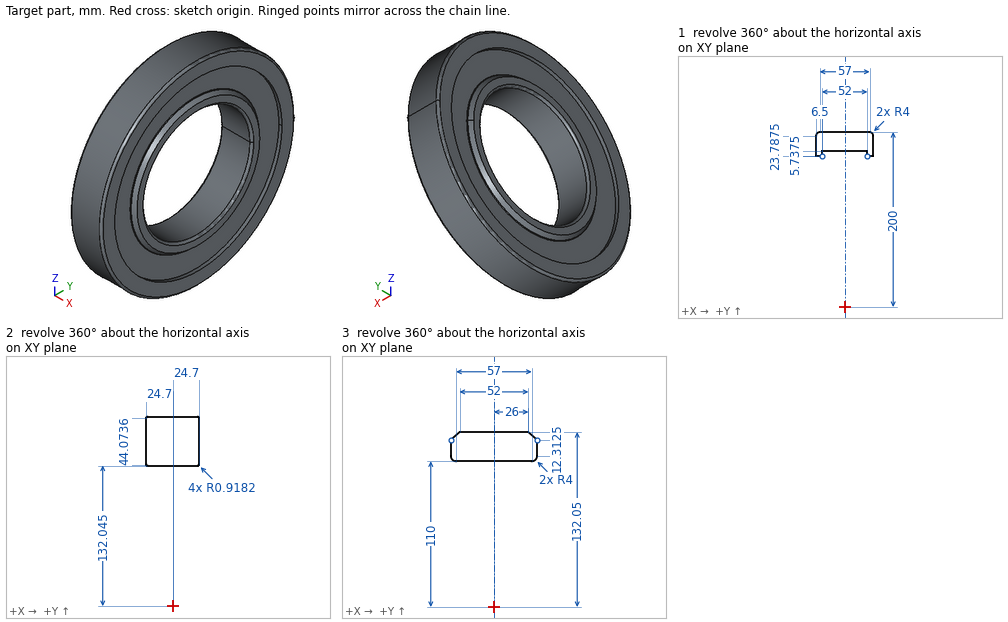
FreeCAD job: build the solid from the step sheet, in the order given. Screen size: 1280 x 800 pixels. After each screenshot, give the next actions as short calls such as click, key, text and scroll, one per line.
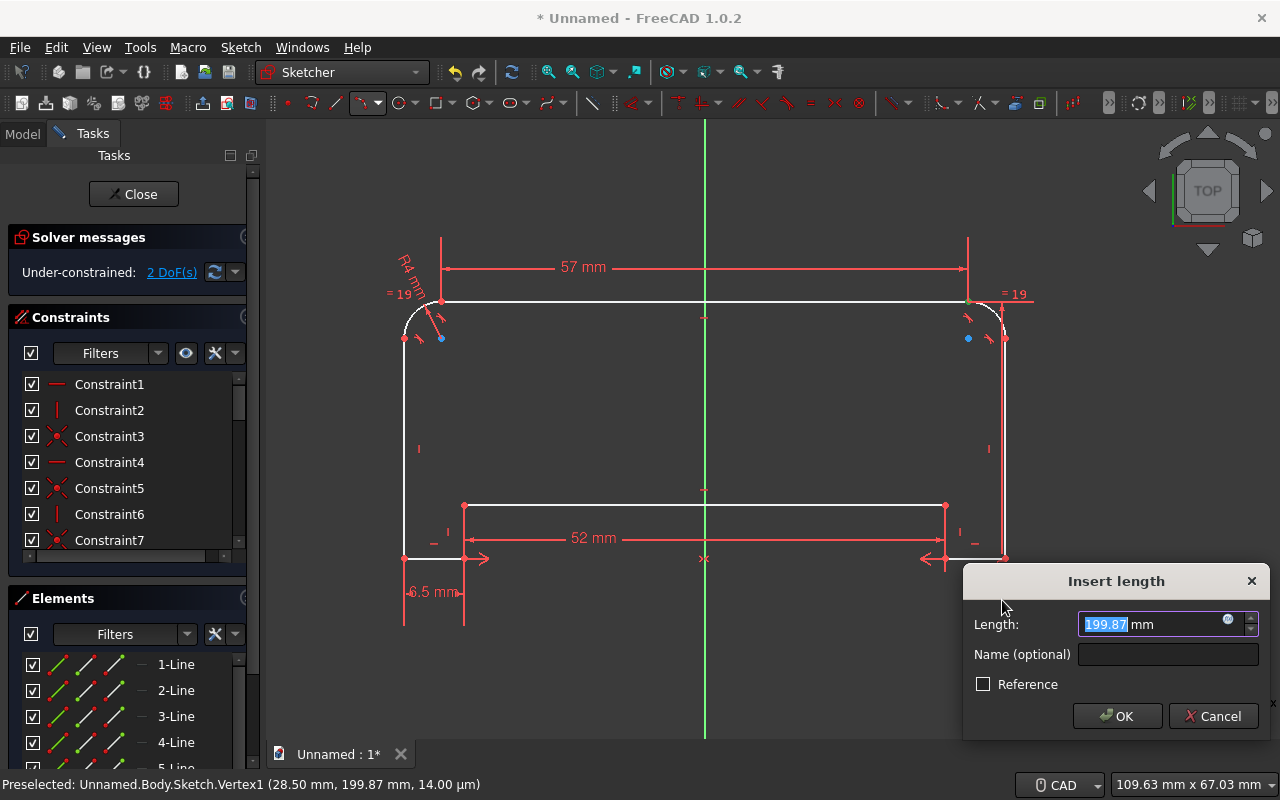
text(200)
key(Return)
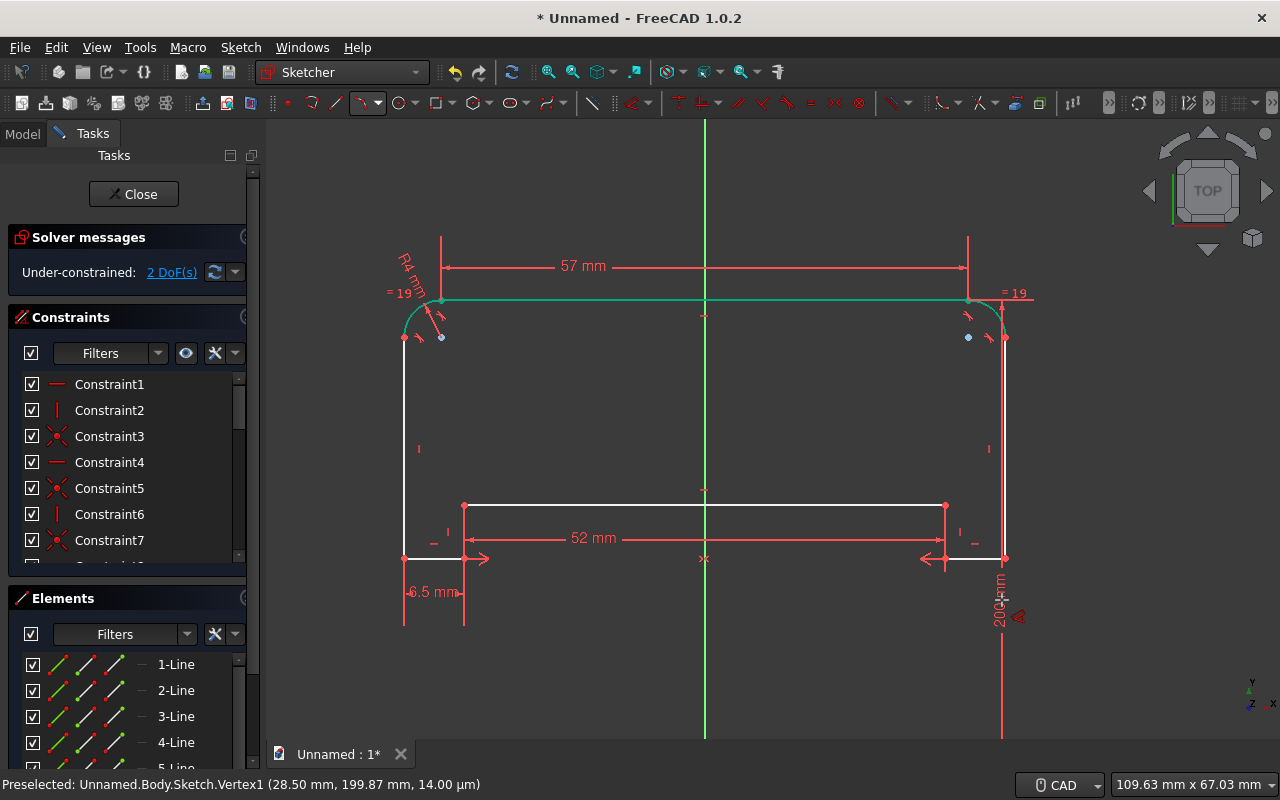
click(464, 543)
click(430, 532)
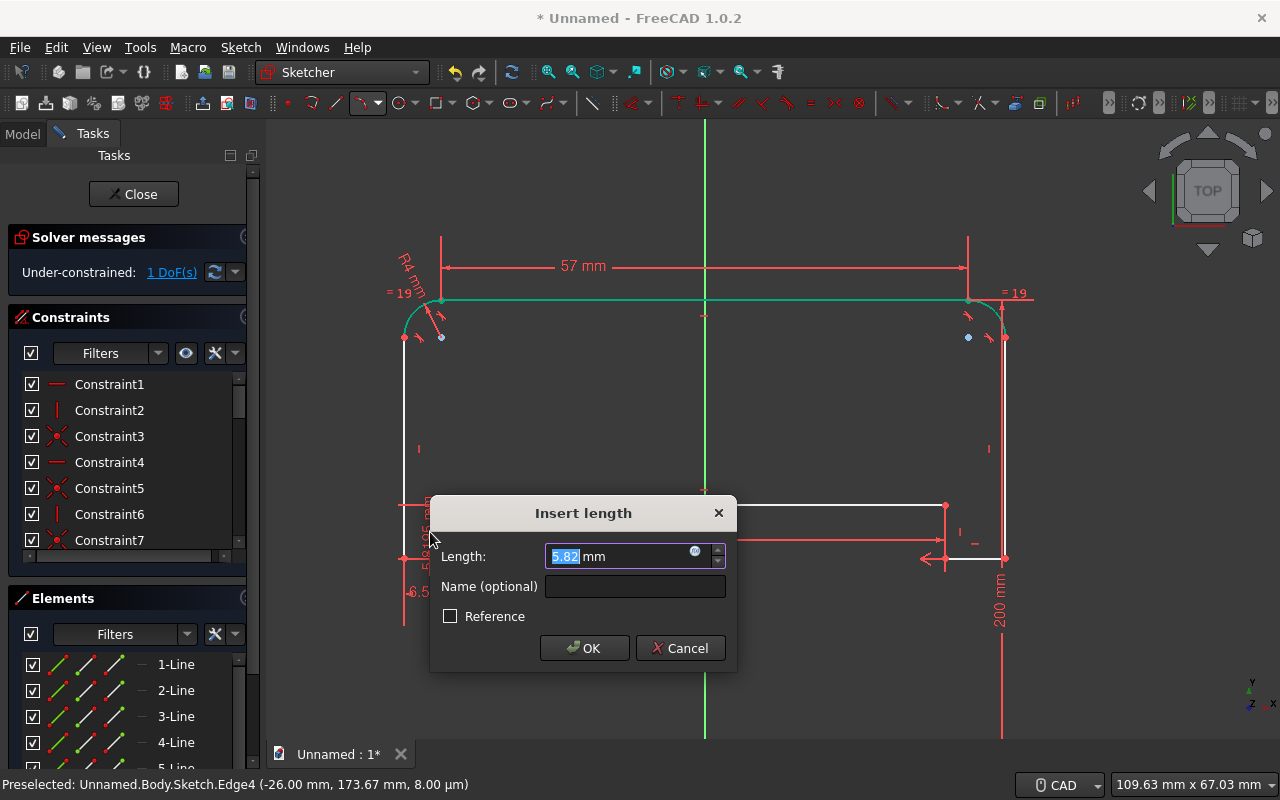
text(5.7375)
key(Return)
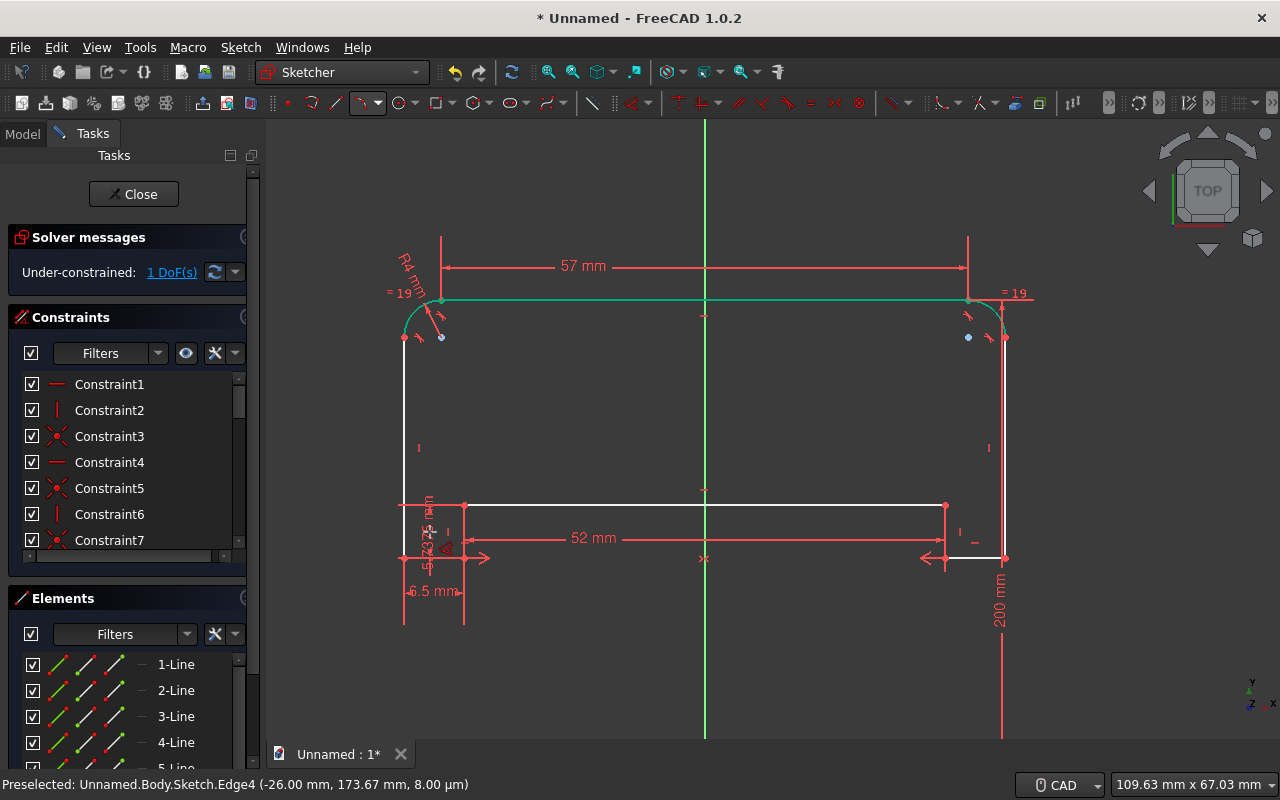
click(404, 404)
click(370, 448)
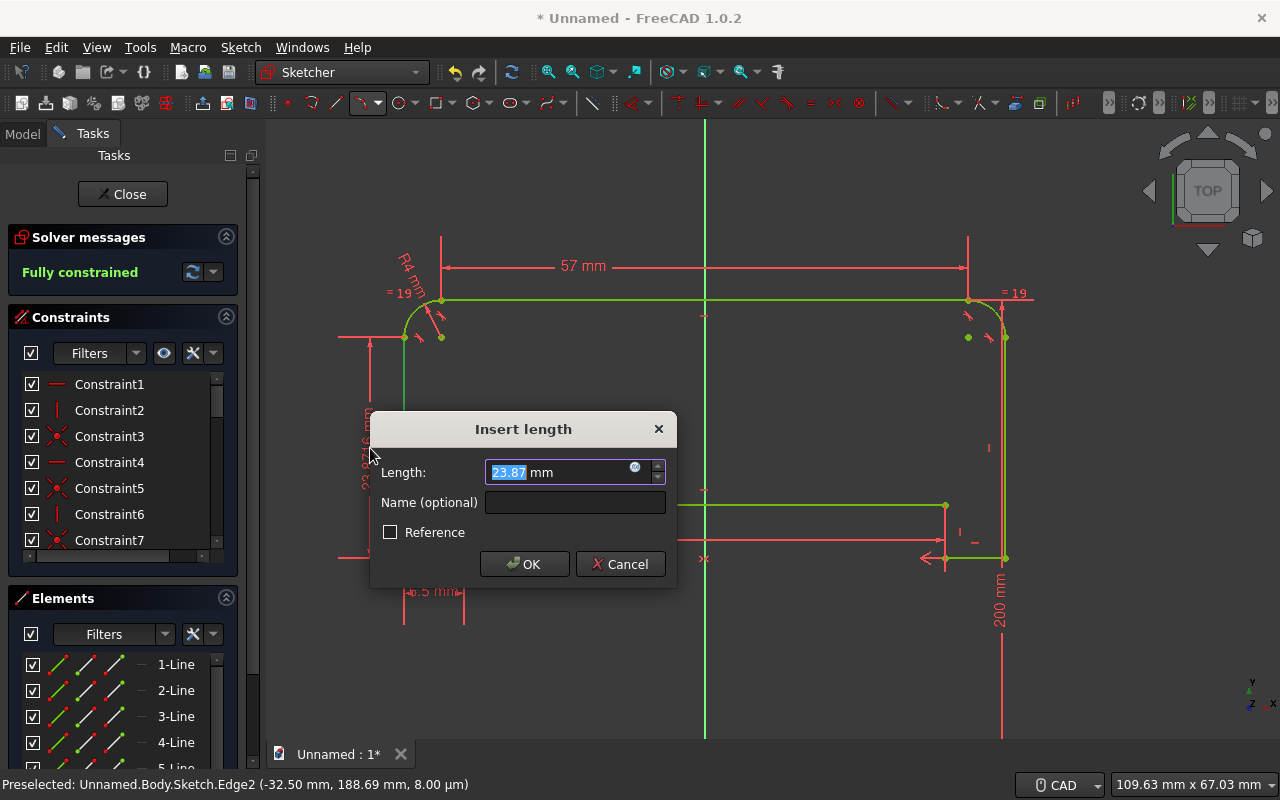
text(23.7875)
key(Return)
key(Escape)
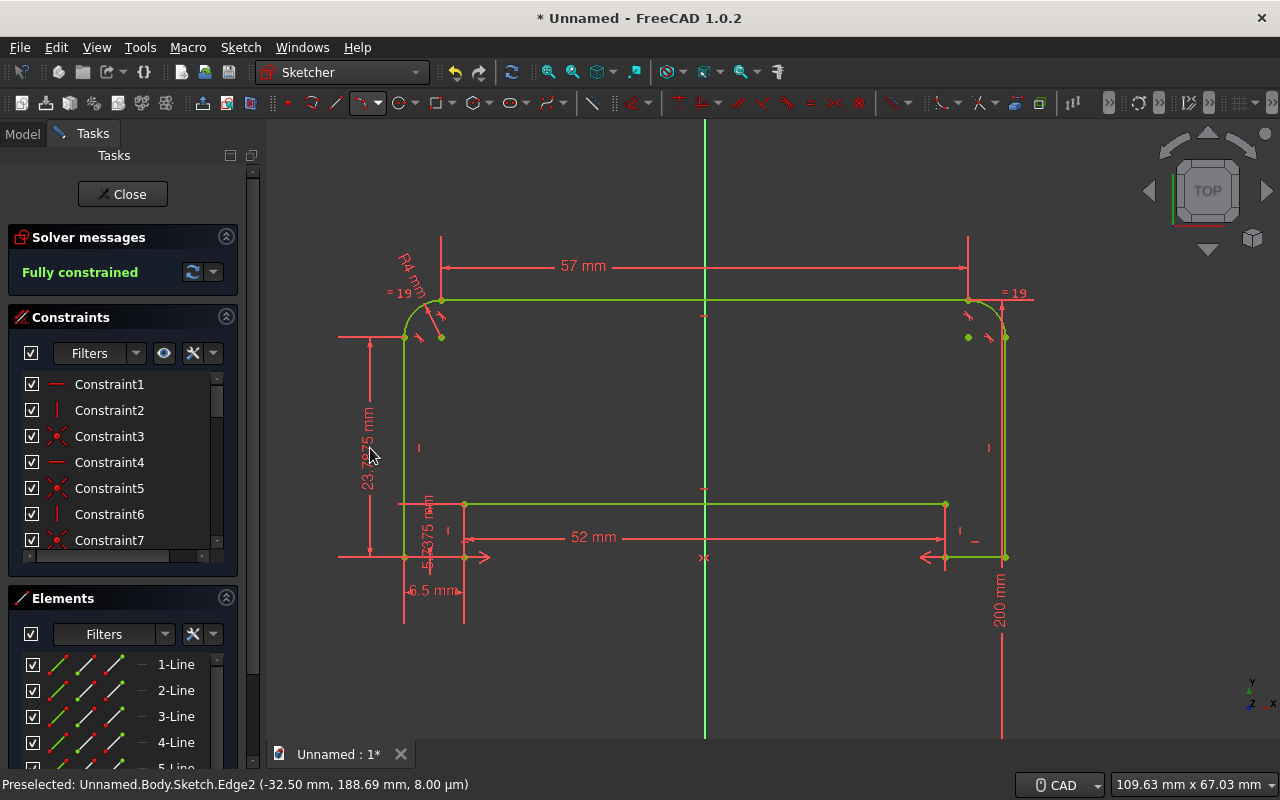
click(123, 194)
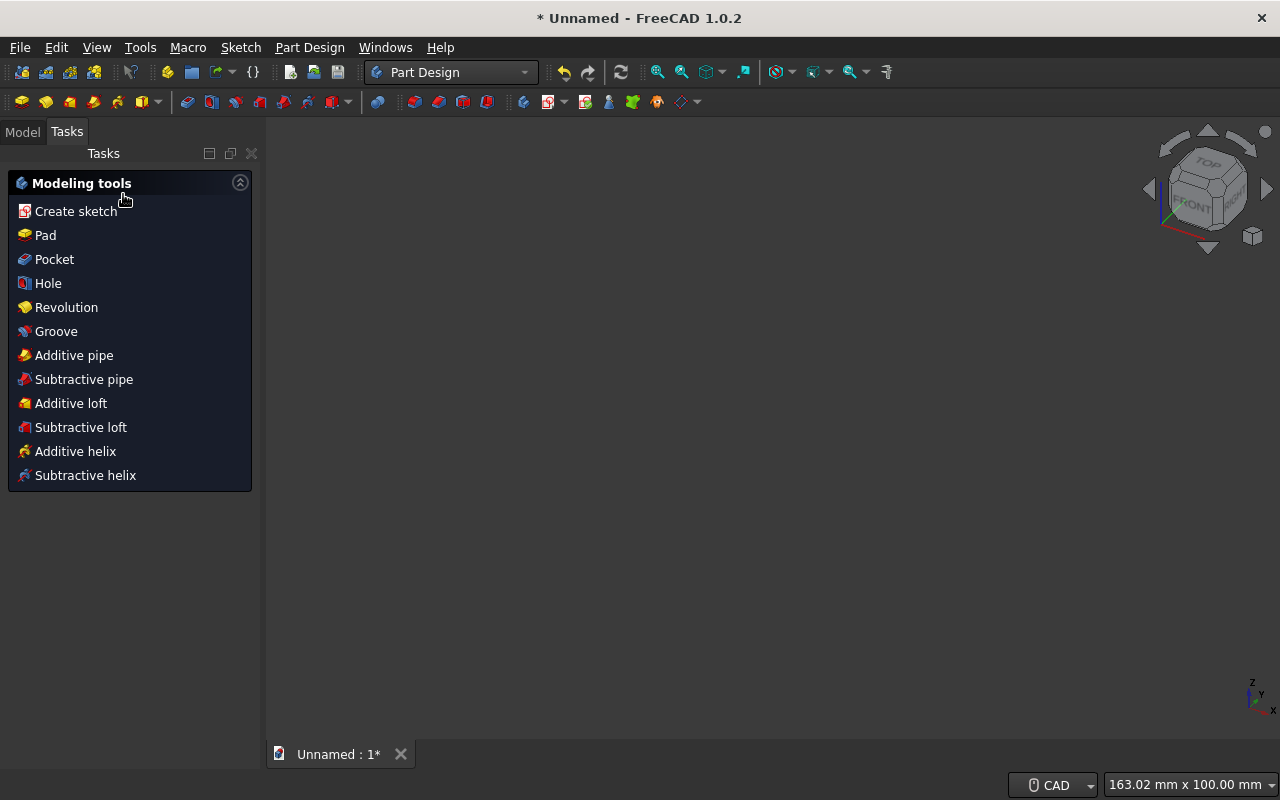
click(46, 102)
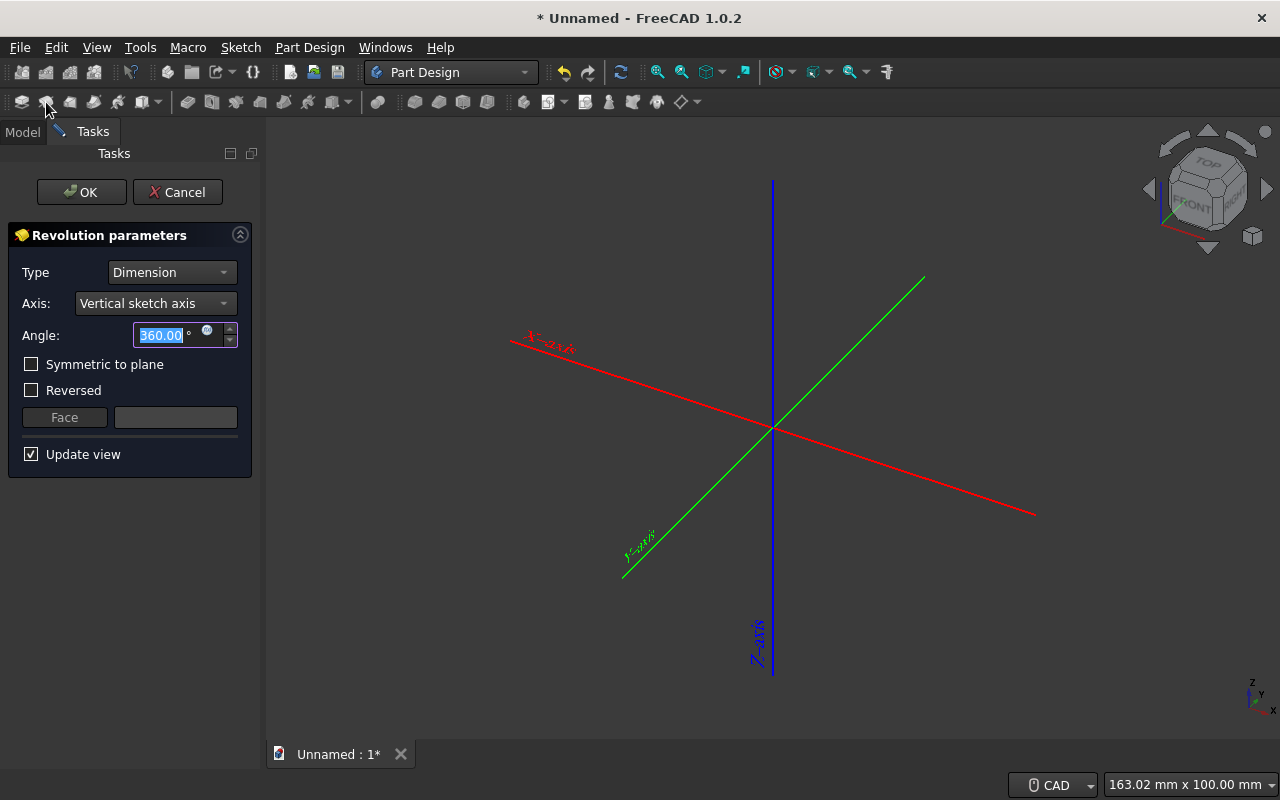
click(156, 304)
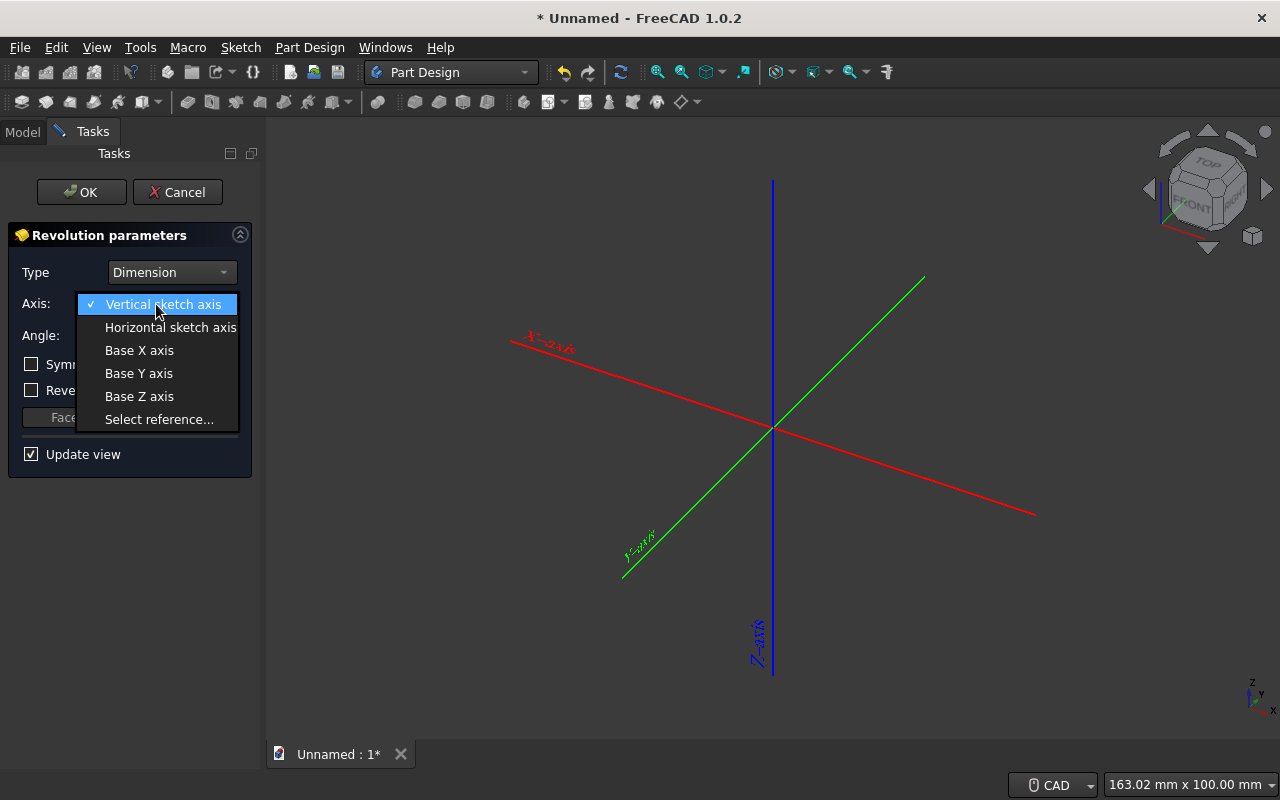
click(156, 328)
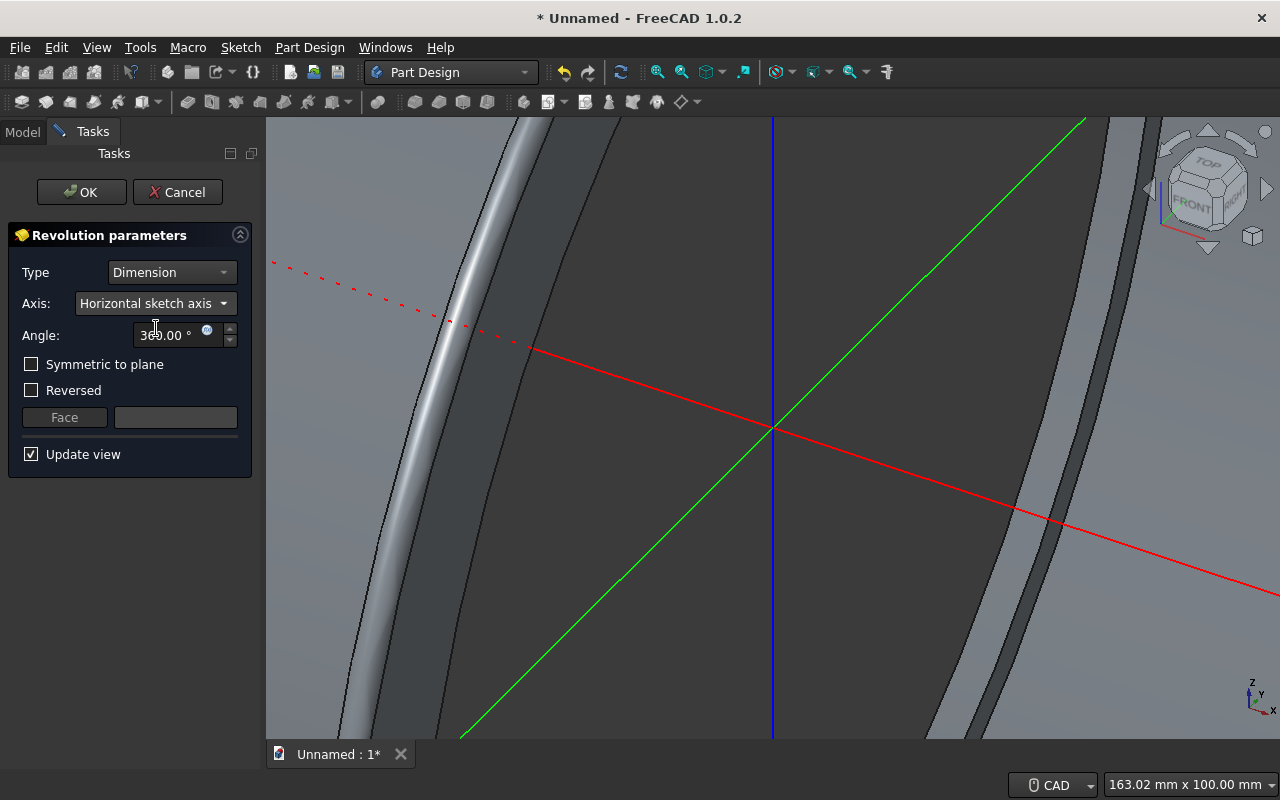
click(82, 192)